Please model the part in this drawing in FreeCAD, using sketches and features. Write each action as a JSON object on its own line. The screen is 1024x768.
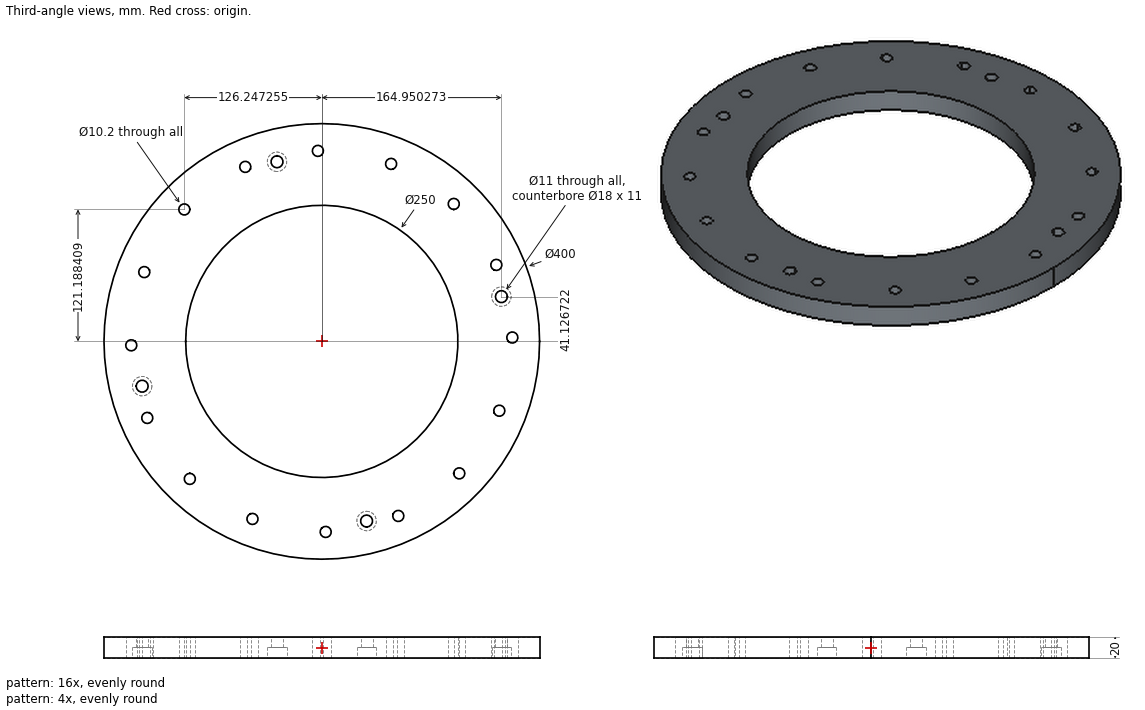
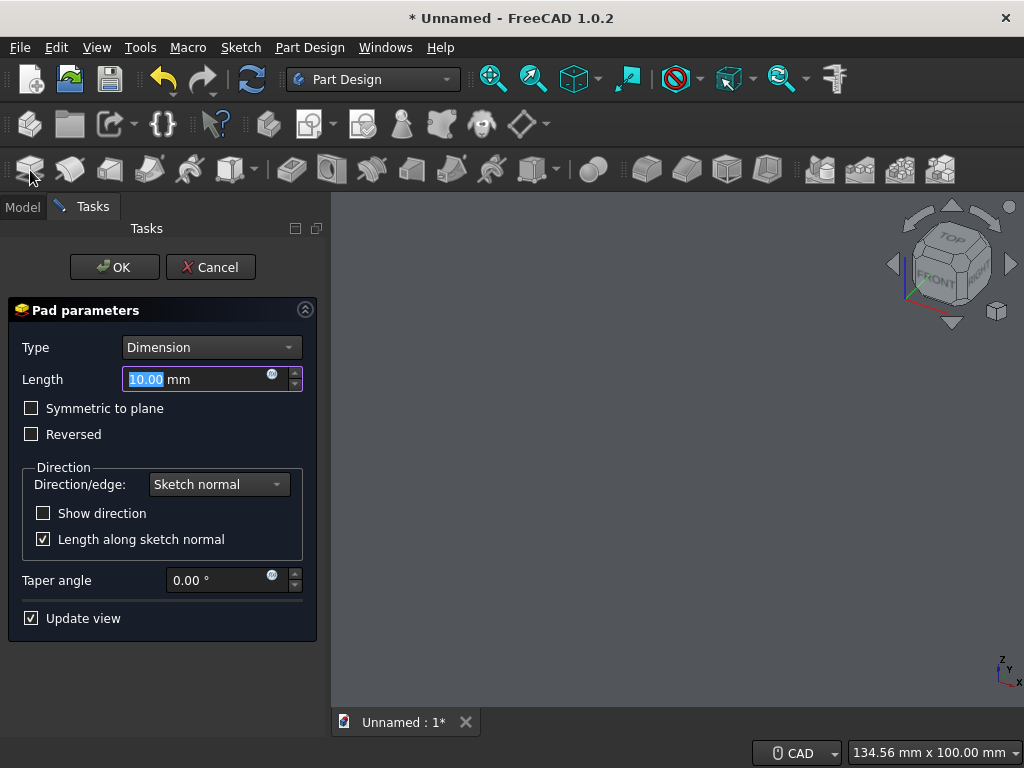
{"action": "type", "text": "20"}
{"action": "key", "text": "Tab"}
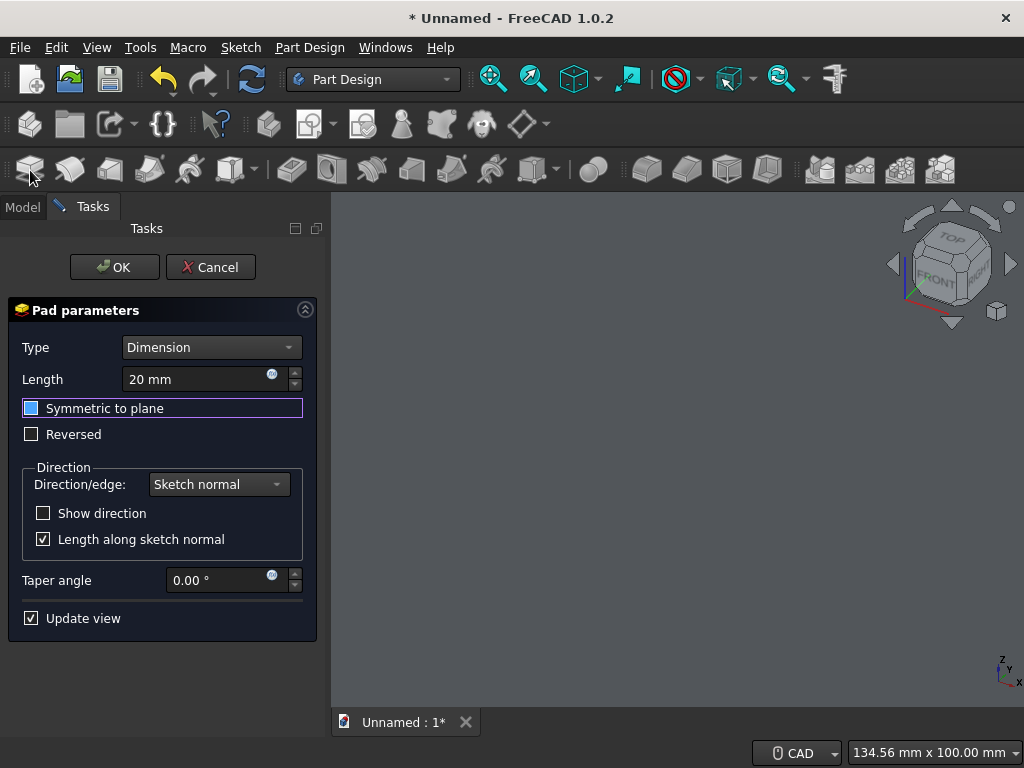
{"action": "left_click", "coordinate": [30, 408]}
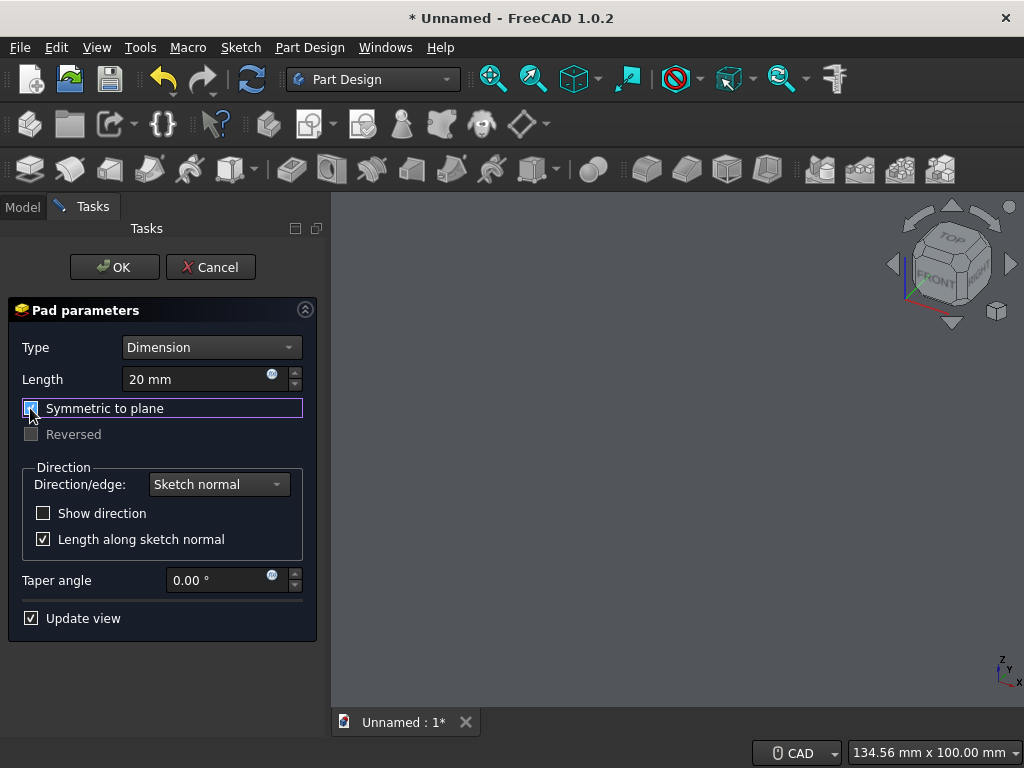
{"action": "left_click", "coordinate": [115, 267]}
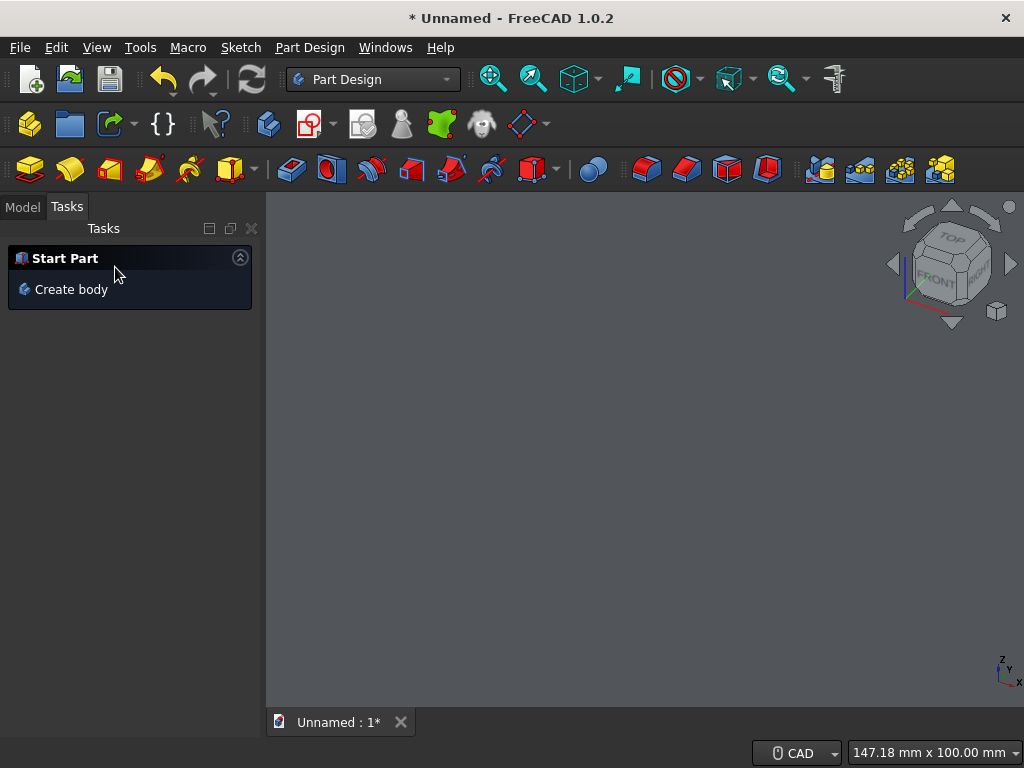
{"action": "left_click", "coordinate": [494, 80]}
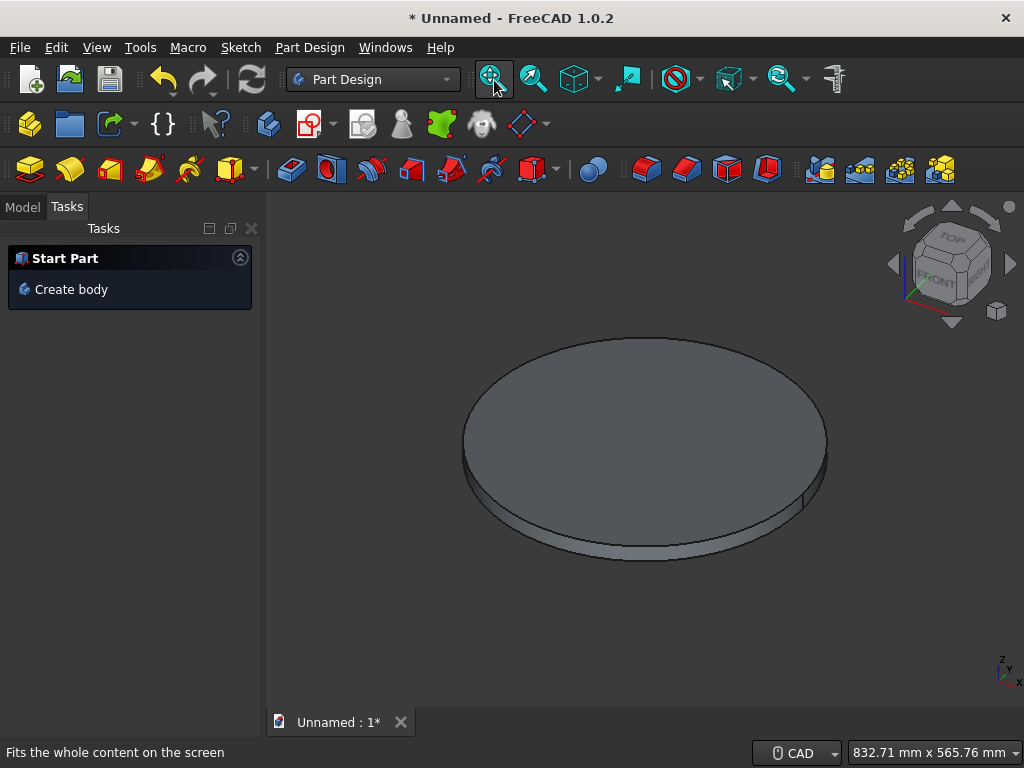
{"action": "key", "text": "5"}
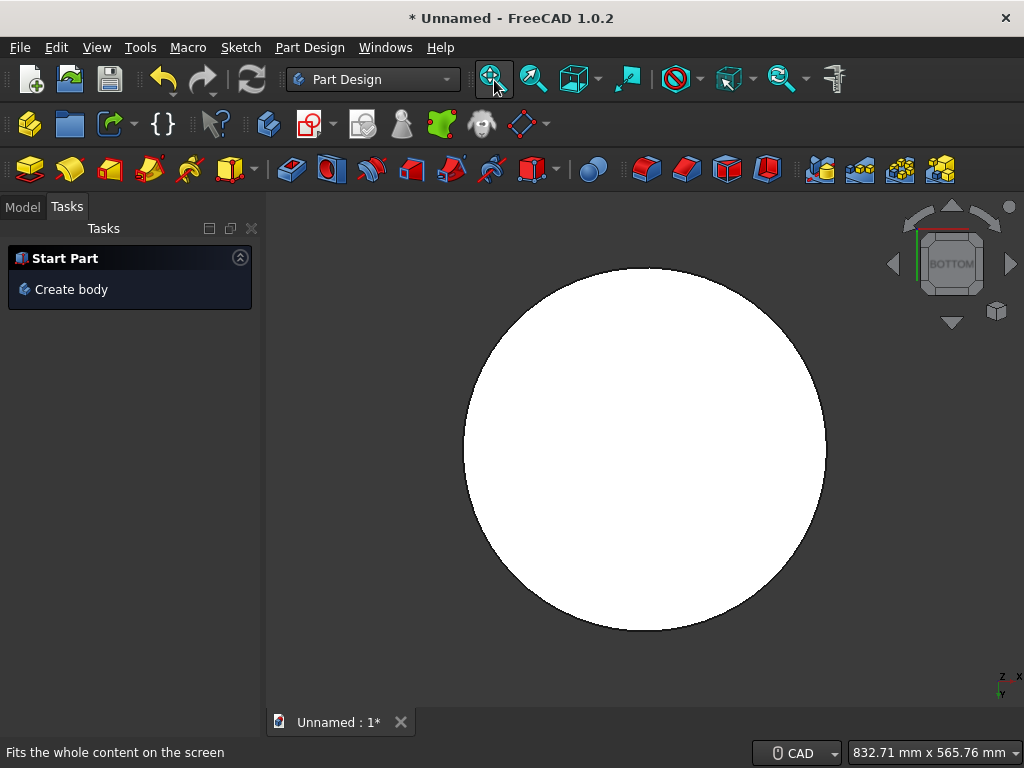
{"action": "left_click", "coordinate": [645, 448]}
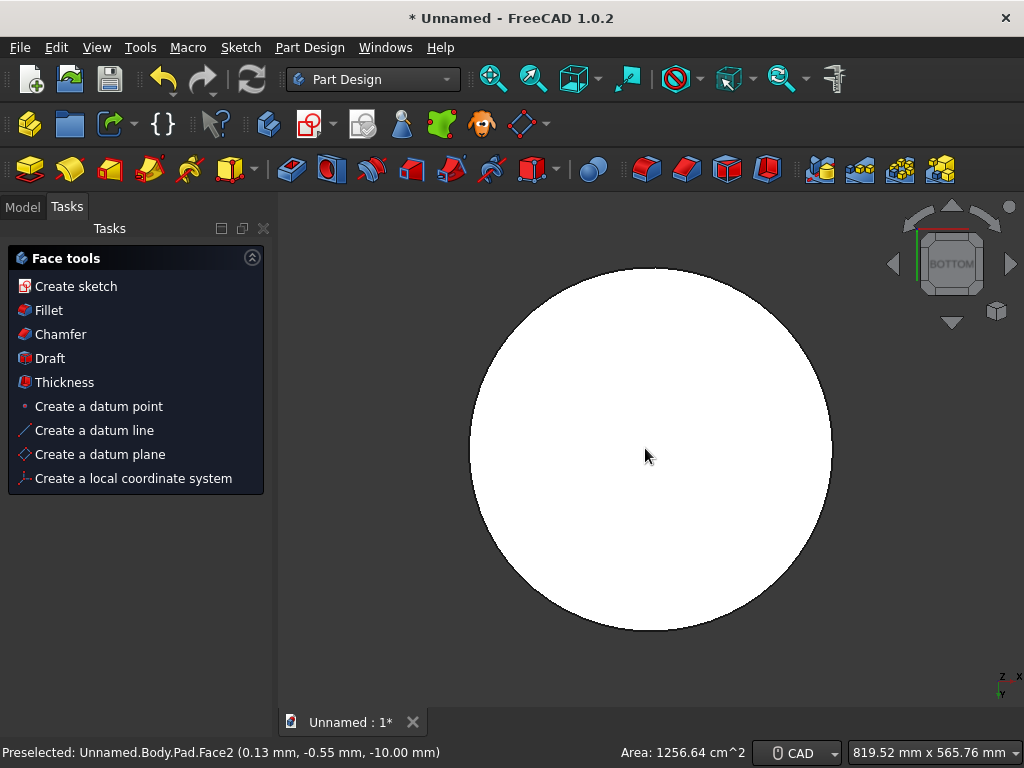
{"action": "left_click", "coordinate": [310, 124]}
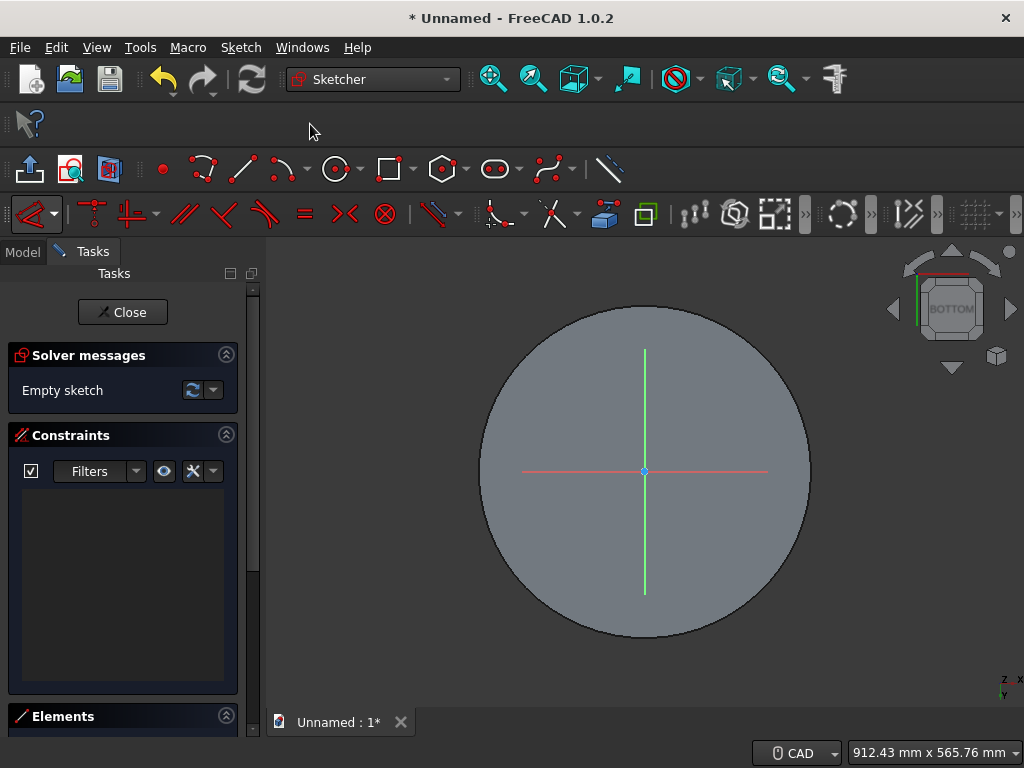
{"action": "scroll", "coordinate": [784, 472], "scroll_direction": "up", "scroll_amount": 2}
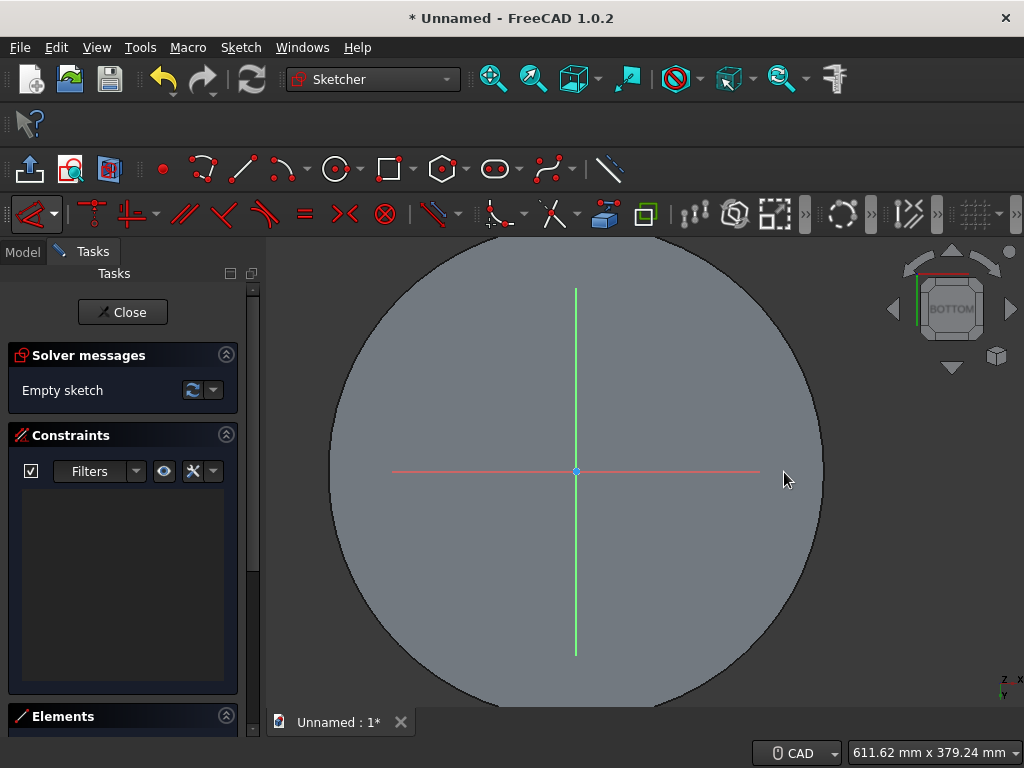
{"action": "left_click", "coordinate": [336, 170]}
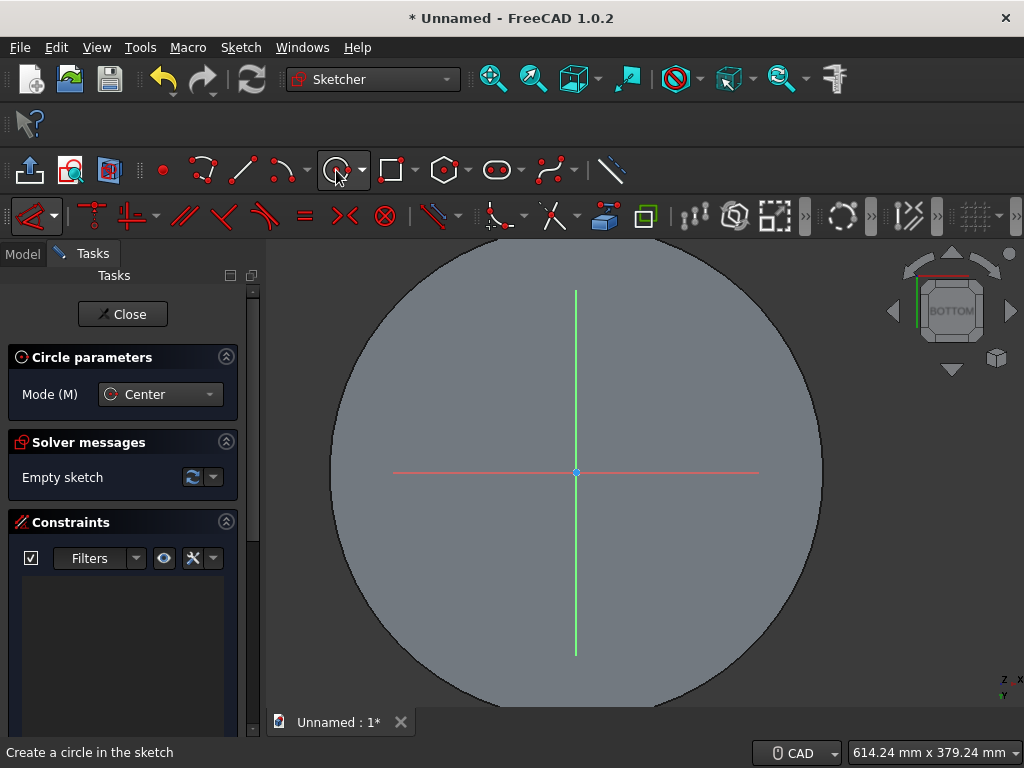
{"action": "left_click", "coordinate": [576, 473]}
{"action": "left_click", "coordinate": [686, 364]}
{"action": "key", "text": "Escape"}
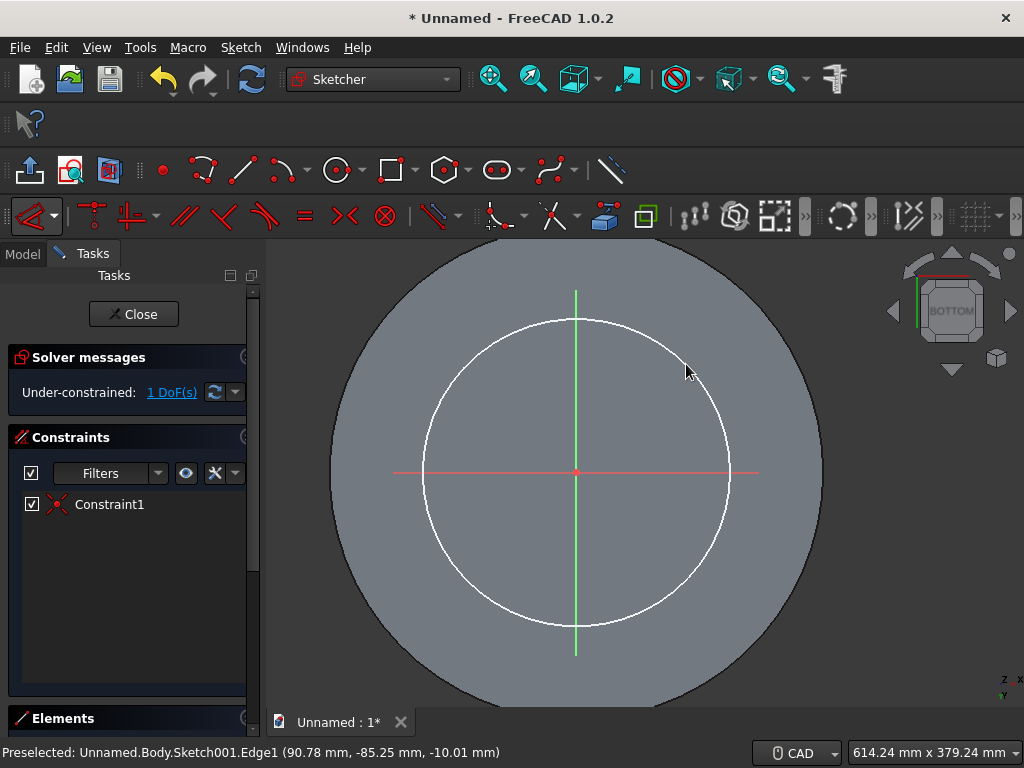
{"action": "left_click", "coordinate": [685, 364]}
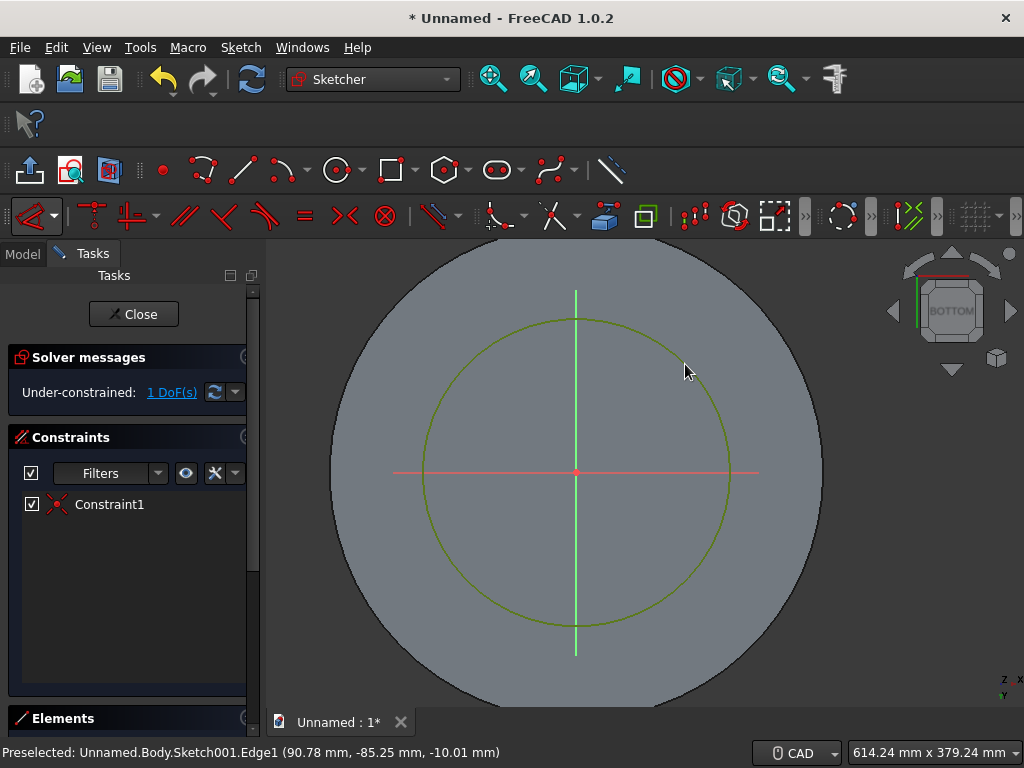
{"action": "key", "text": "k o"}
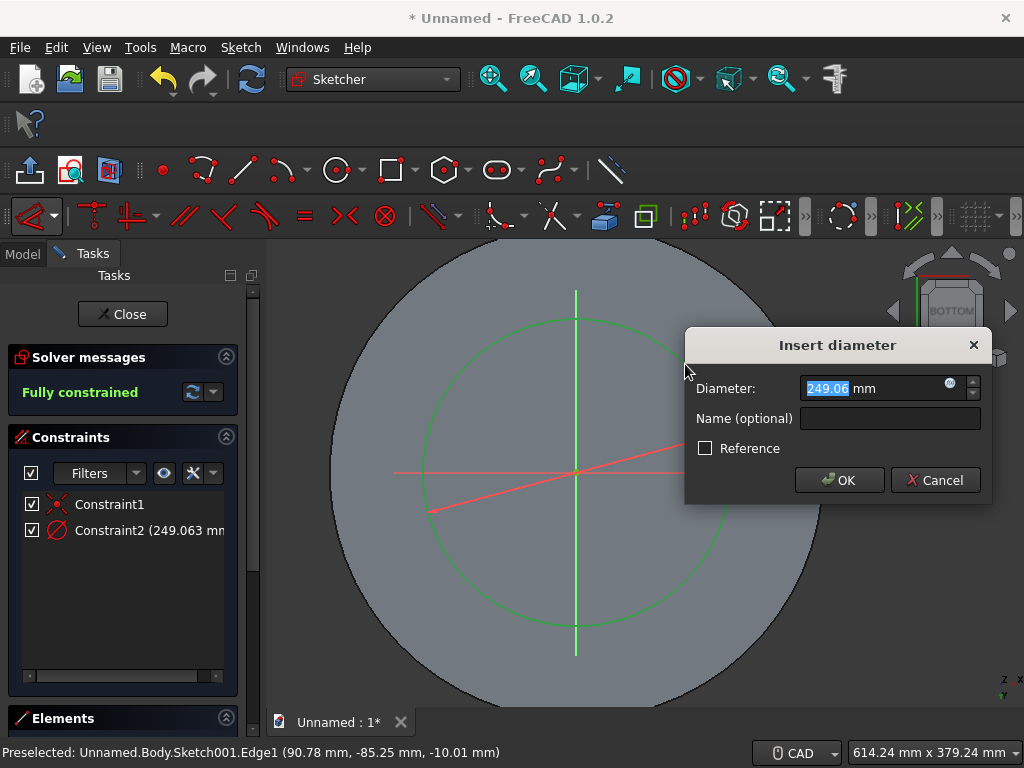
{"action": "type", "text": "250"}
{"action": "key", "text": "Return"}